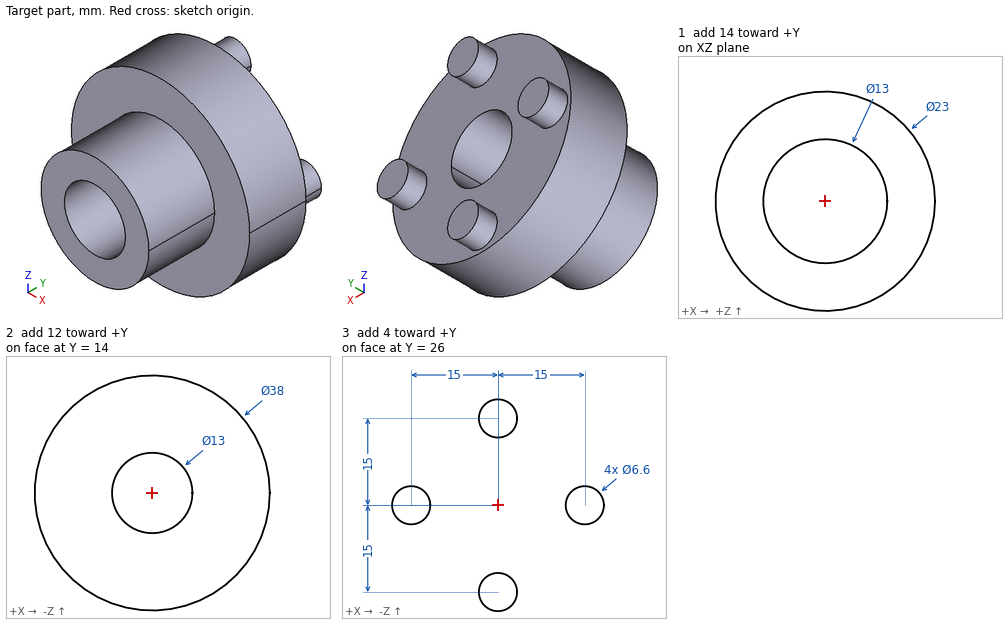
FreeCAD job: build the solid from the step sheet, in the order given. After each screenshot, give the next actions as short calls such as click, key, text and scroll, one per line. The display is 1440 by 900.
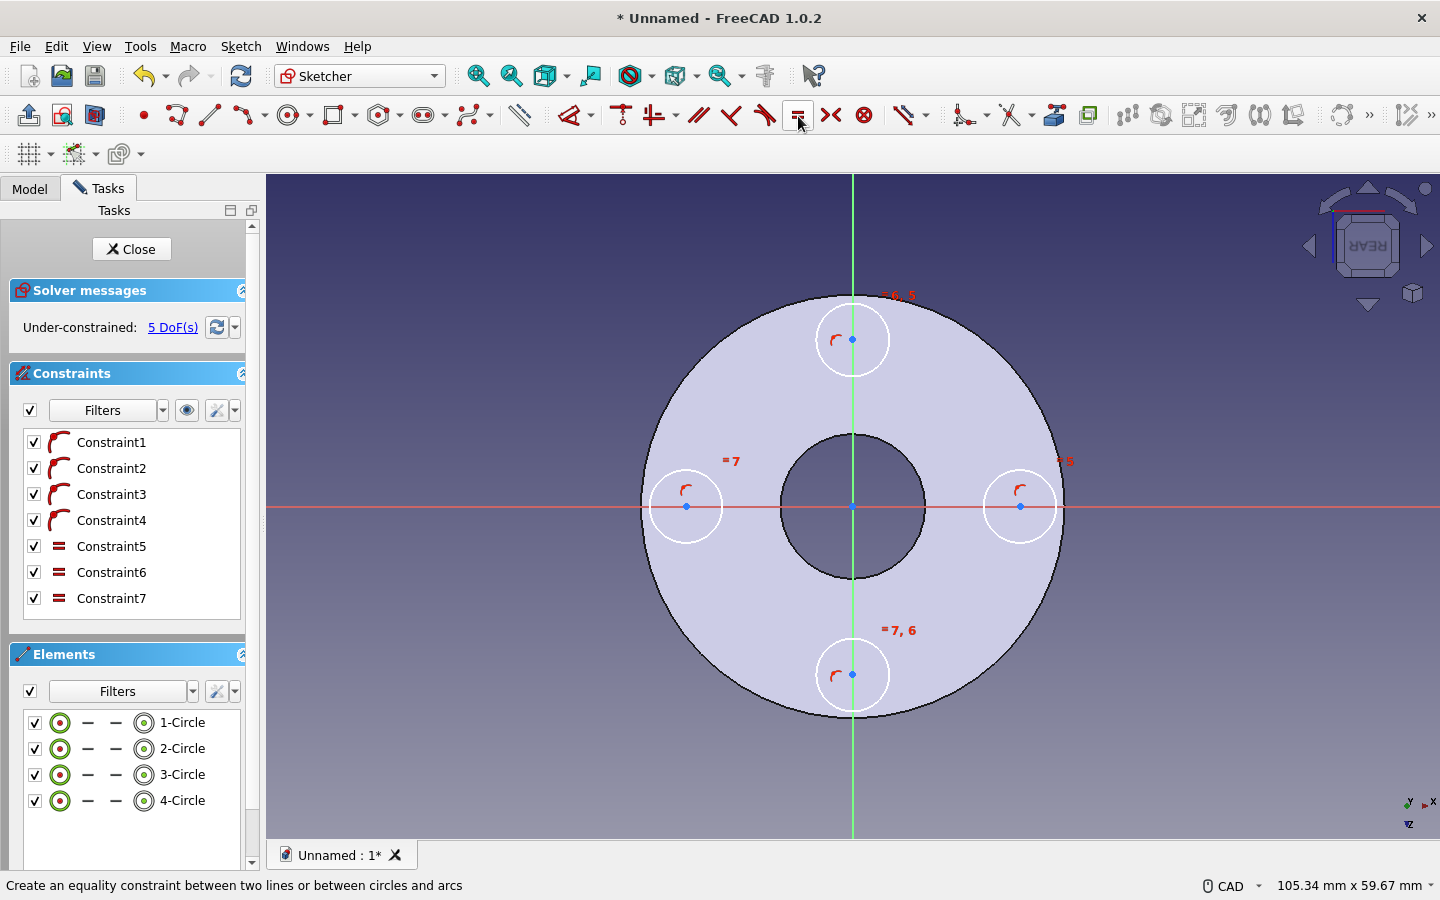
key(d)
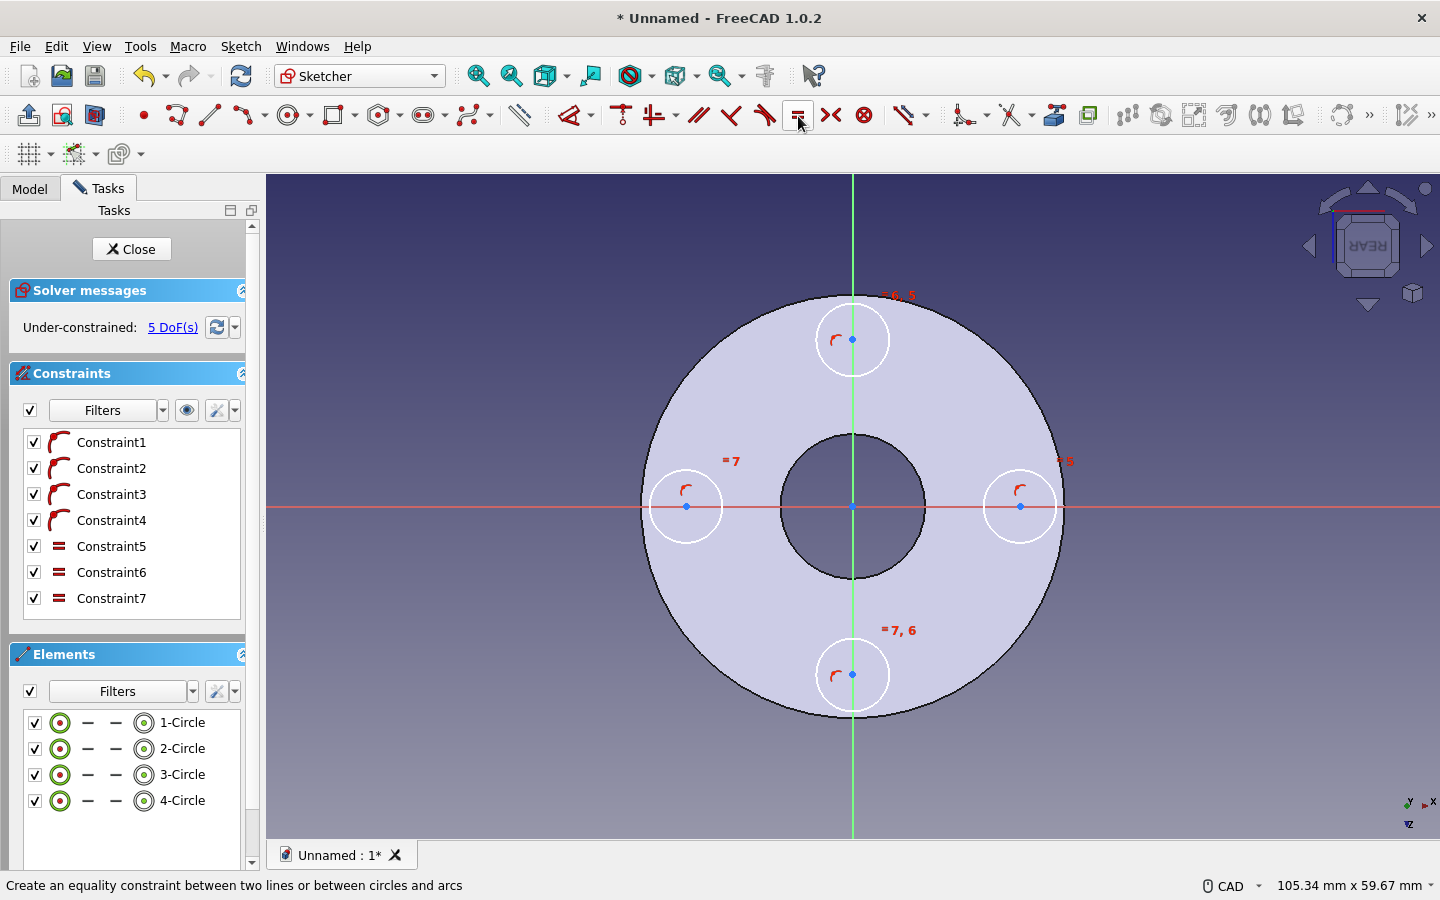
click(1046, 481)
click(1069, 459)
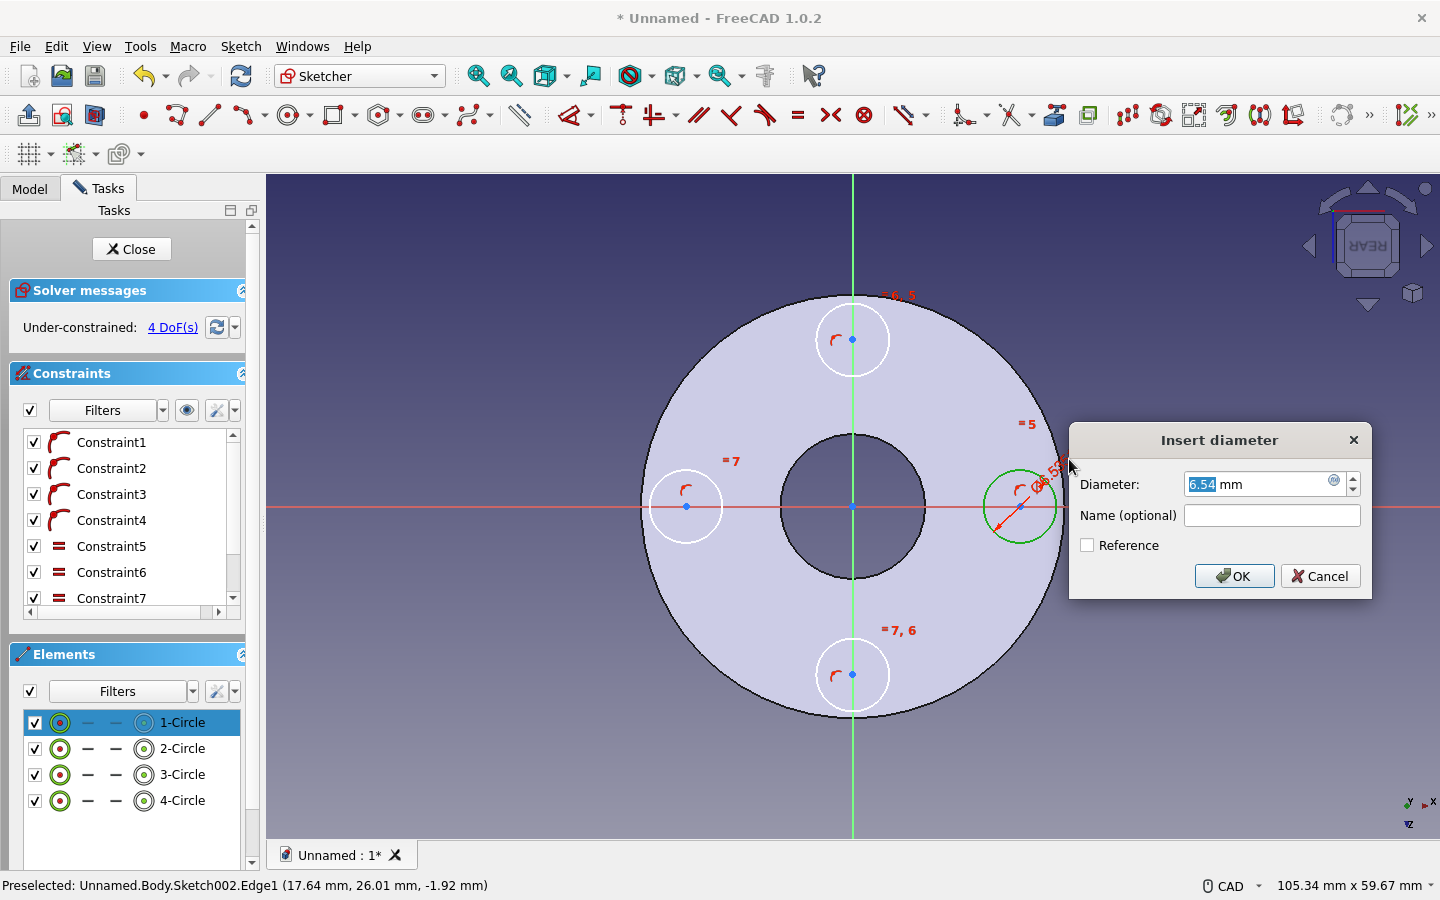
text(6.6)
key(Return)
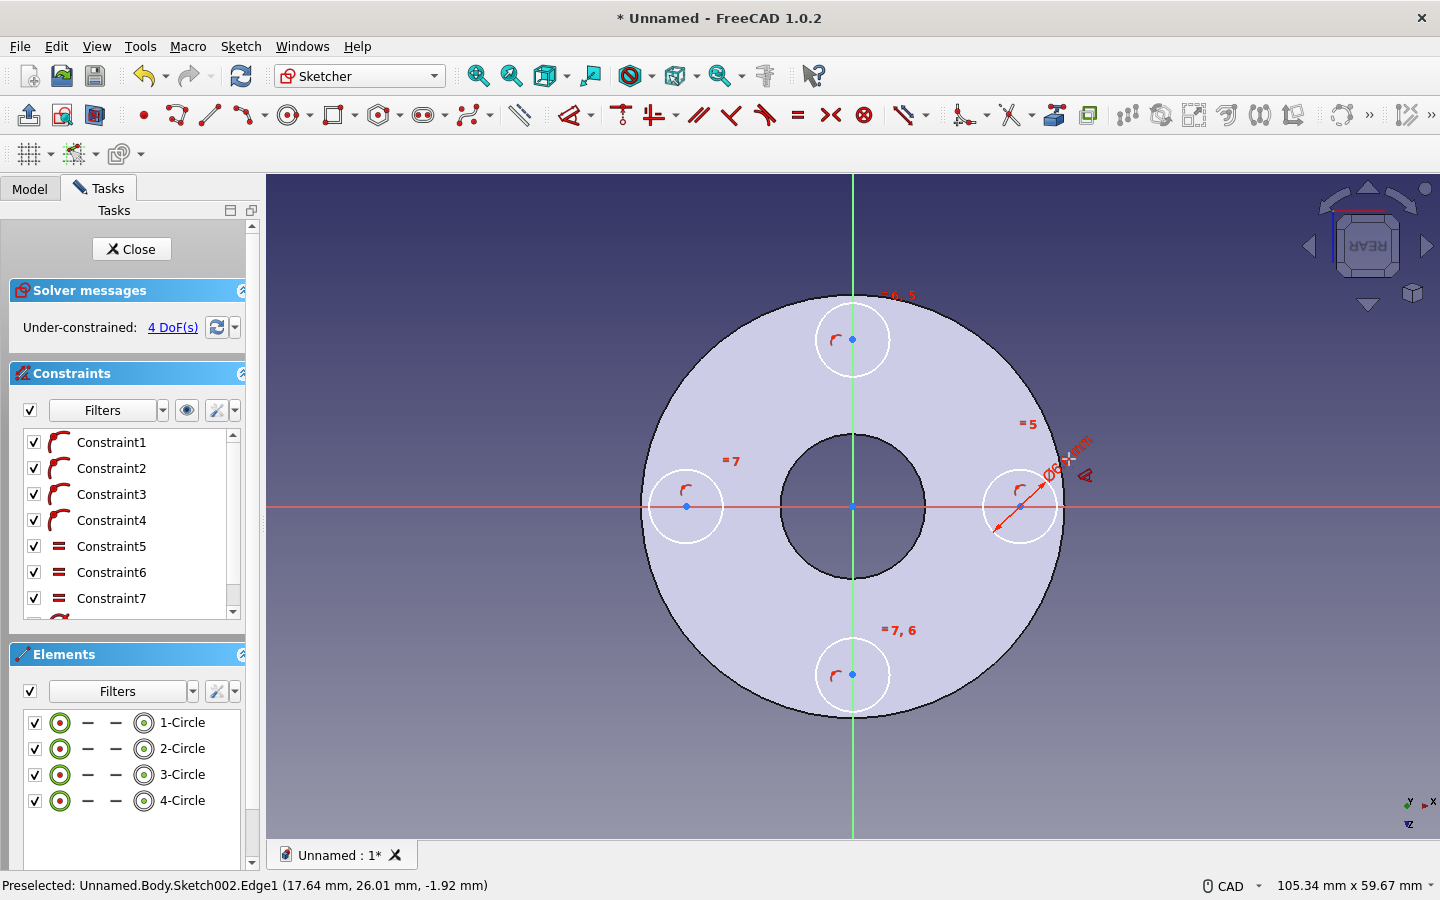
click(1020, 506)
click(936, 540)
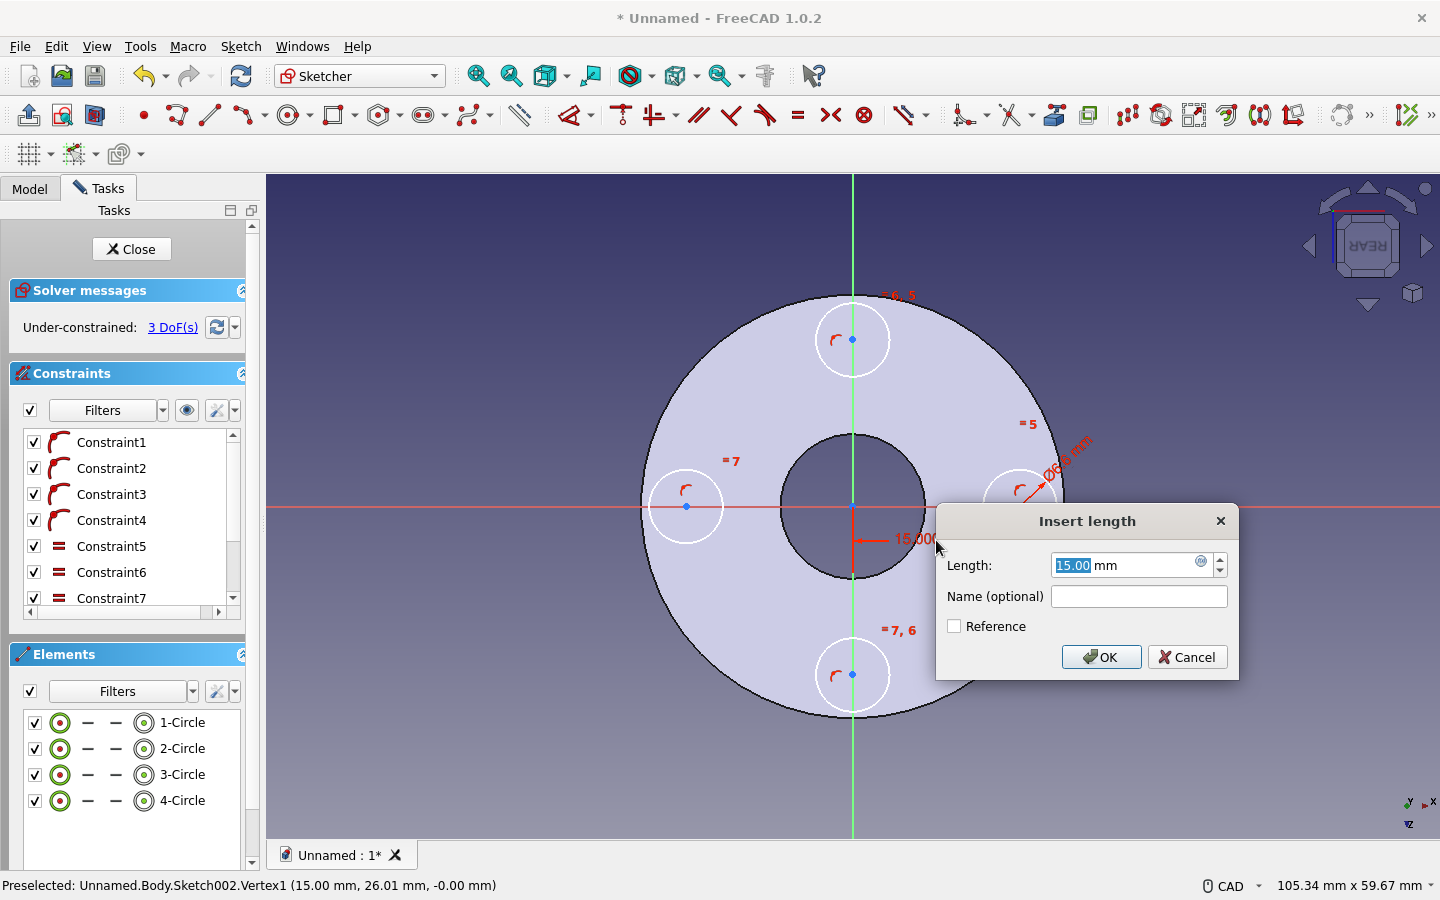
text(15)
key(Return)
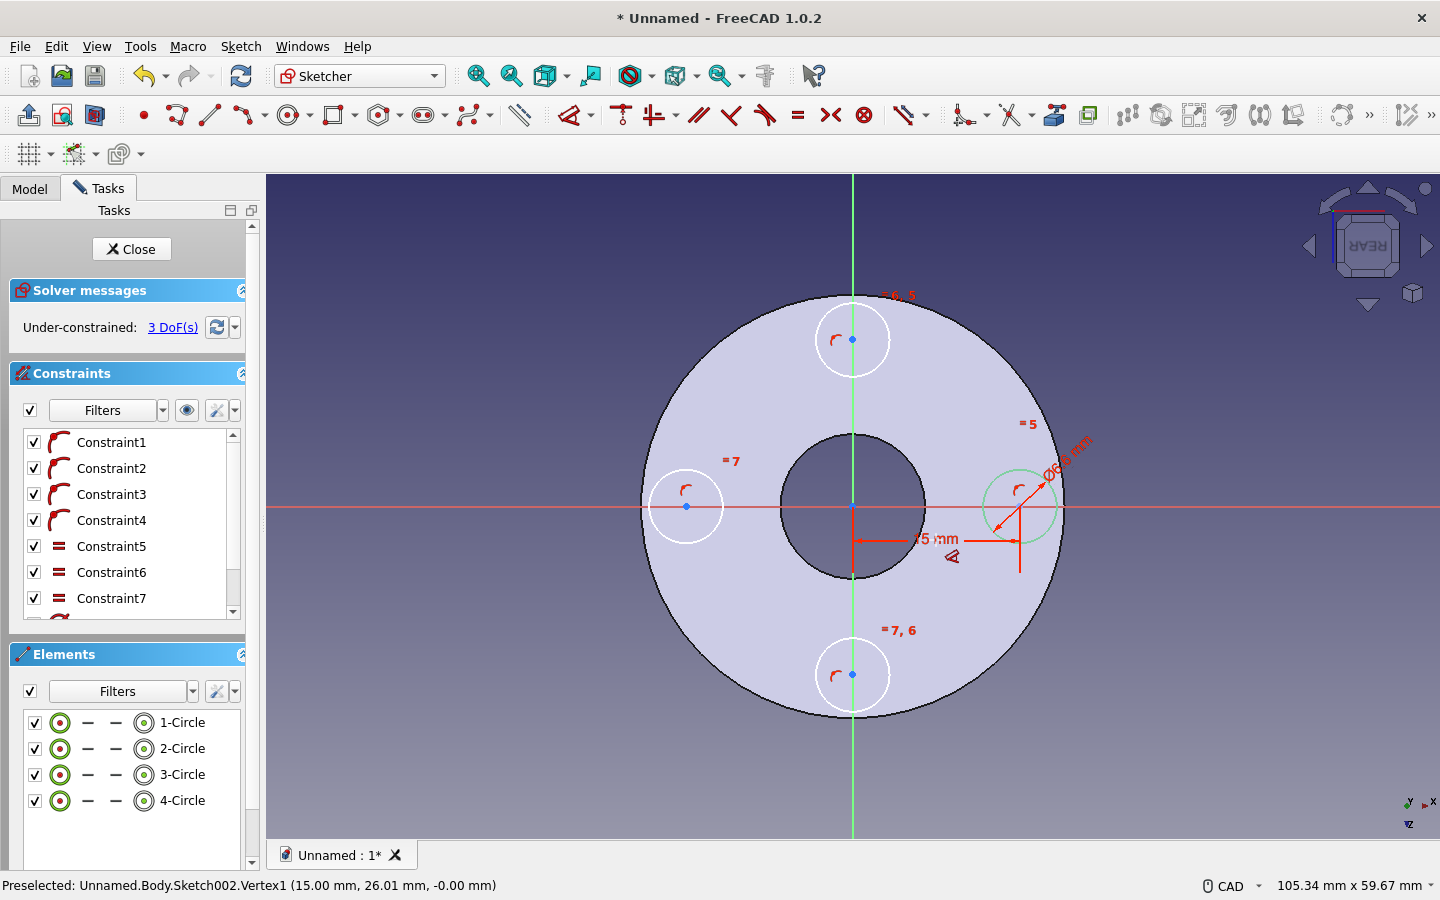
click(853, 340)
click(887, 423)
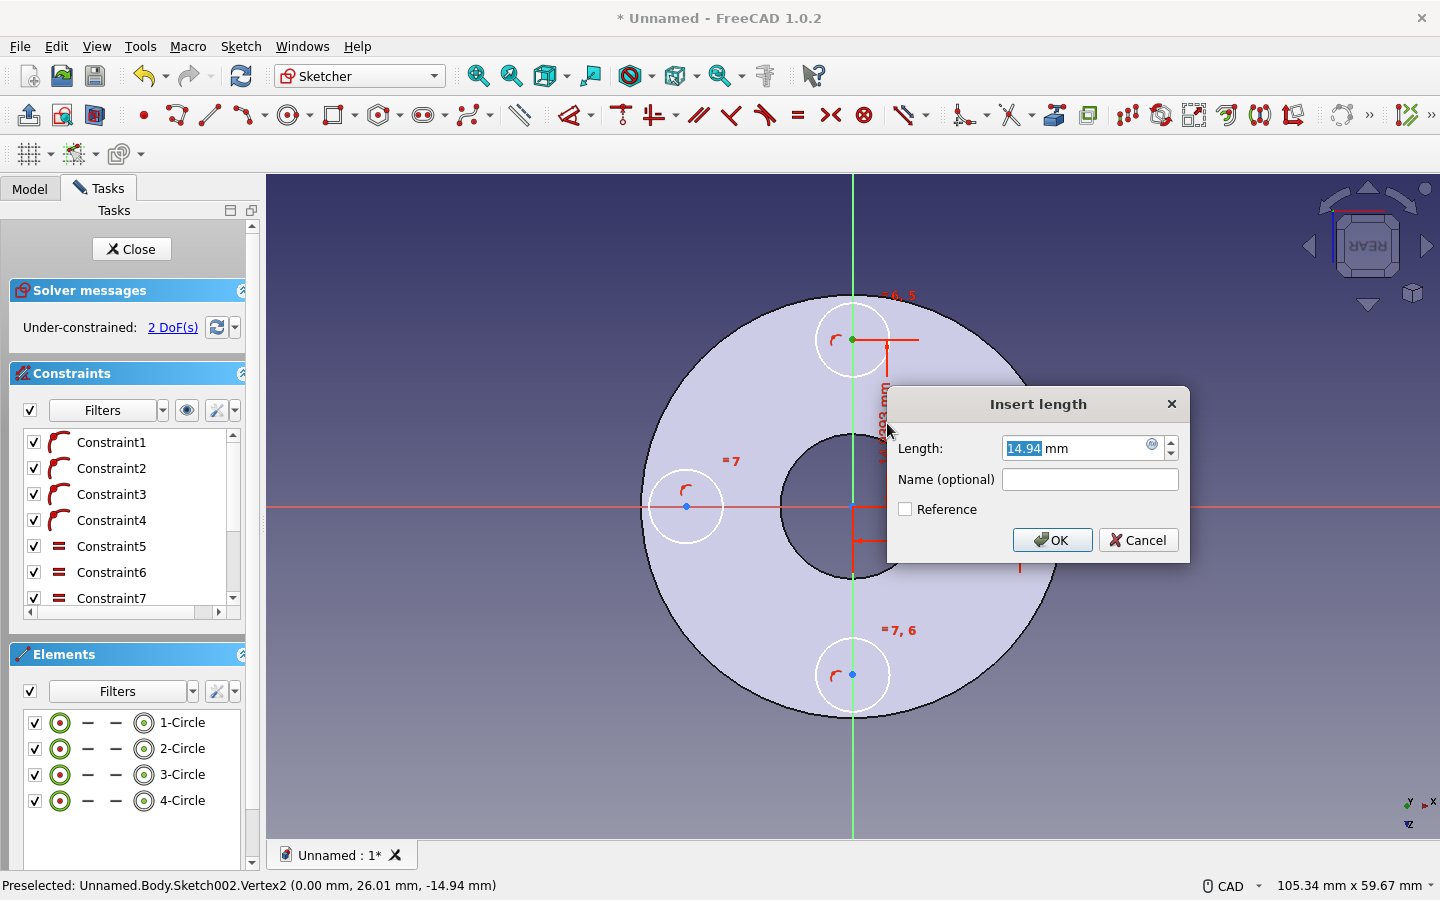
text(15)
key(Return)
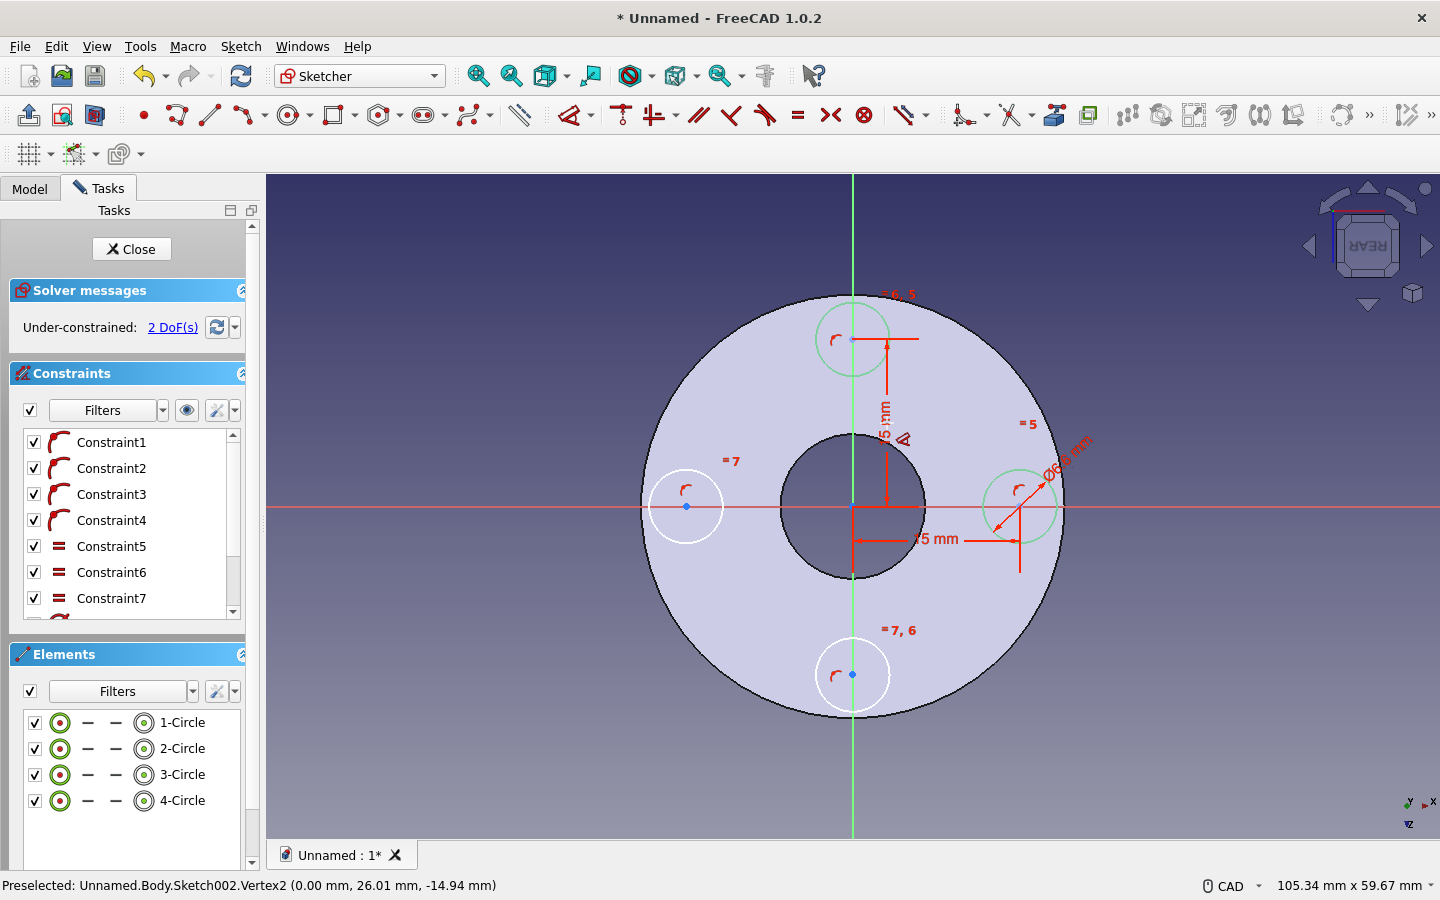
click(853, 675)
click(887, 591)